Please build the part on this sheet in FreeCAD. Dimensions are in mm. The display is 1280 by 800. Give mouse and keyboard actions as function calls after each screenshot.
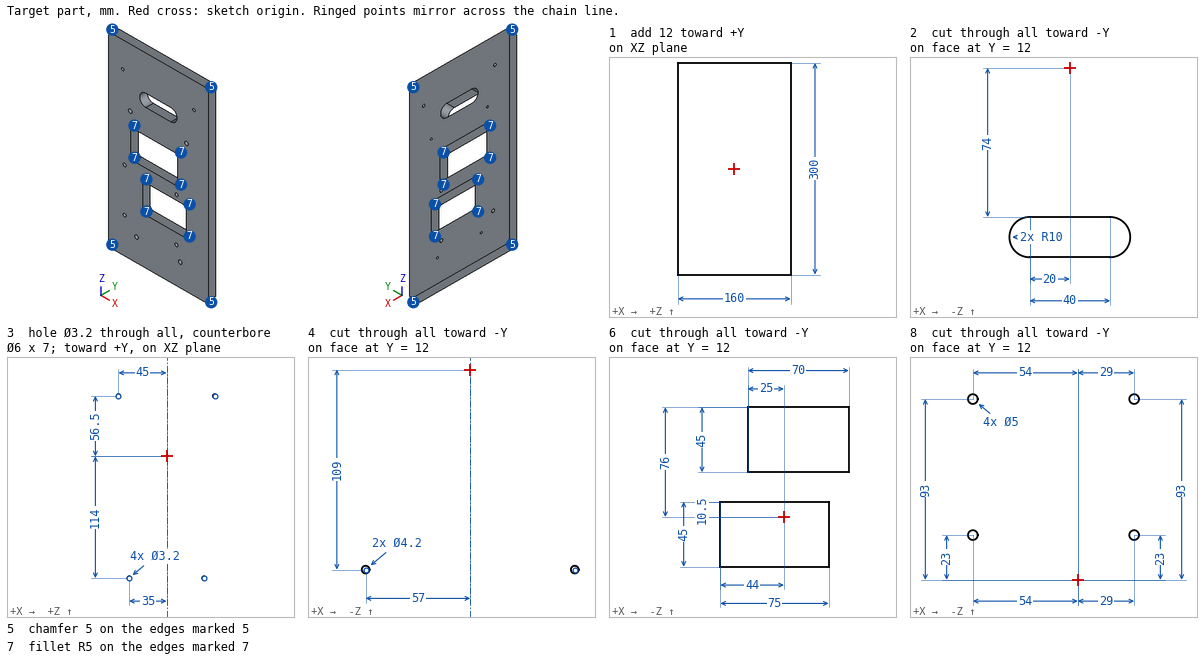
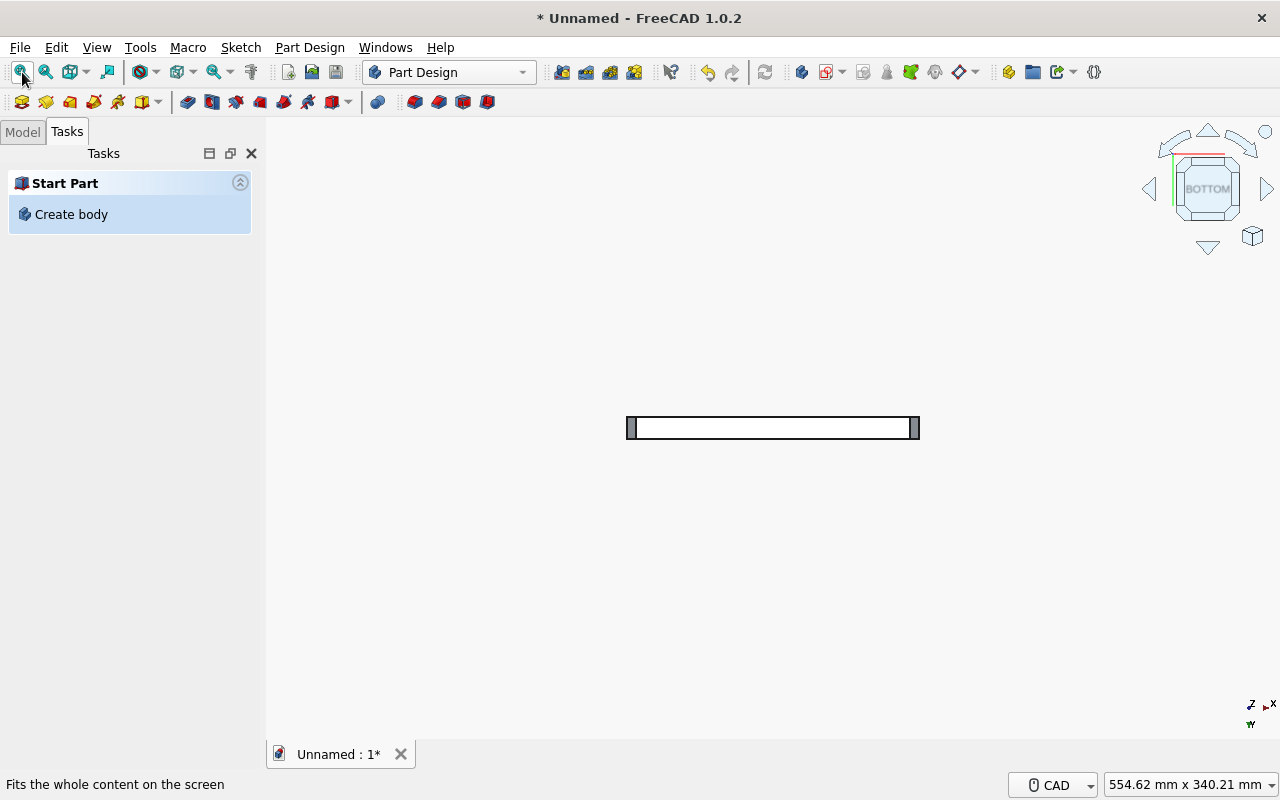
click(22, 72)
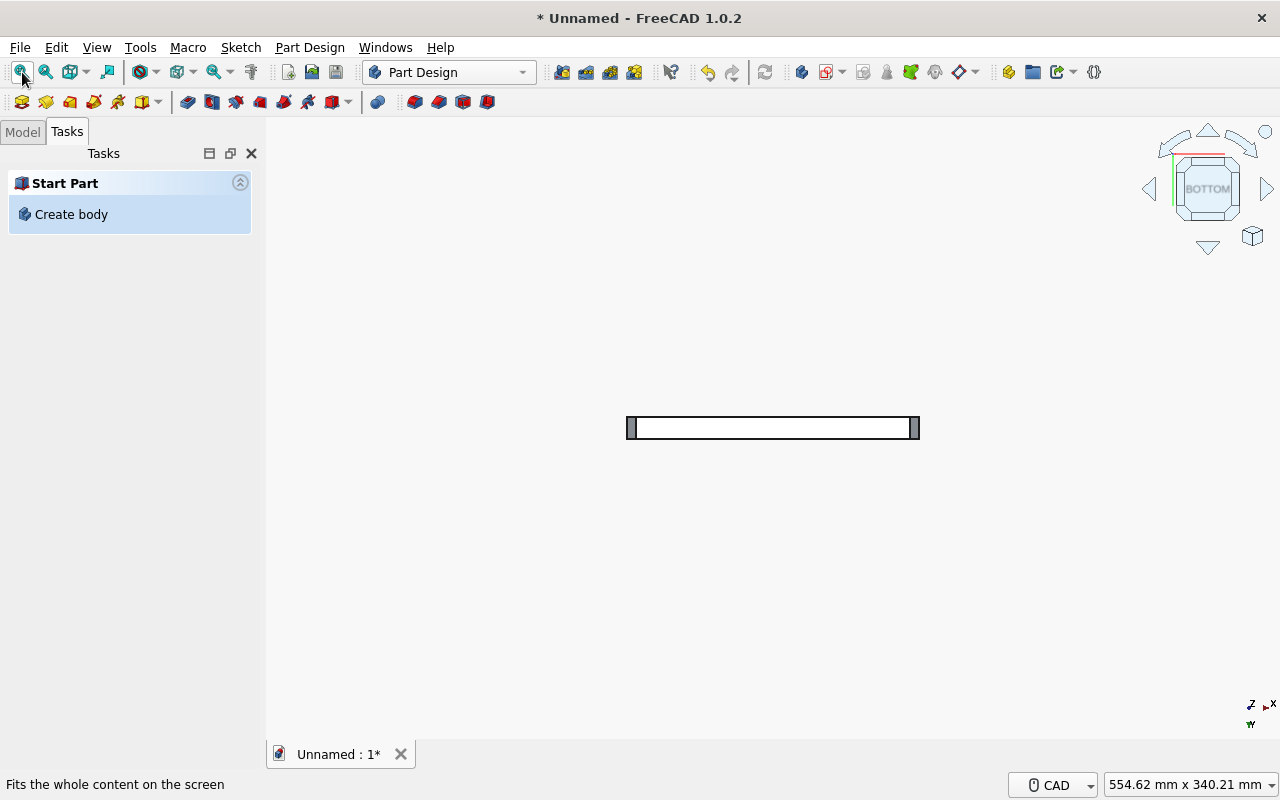
scroll(830, 427, up, 4)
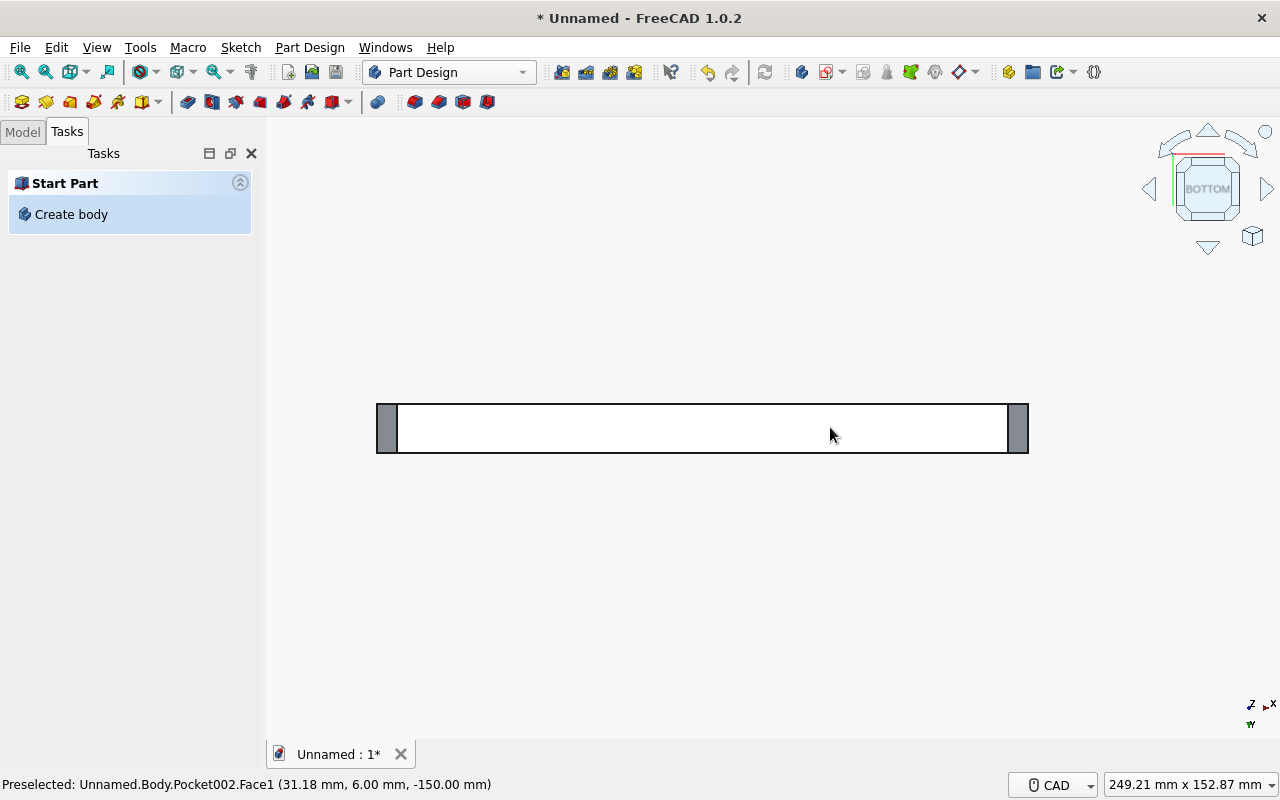
click(22, 72)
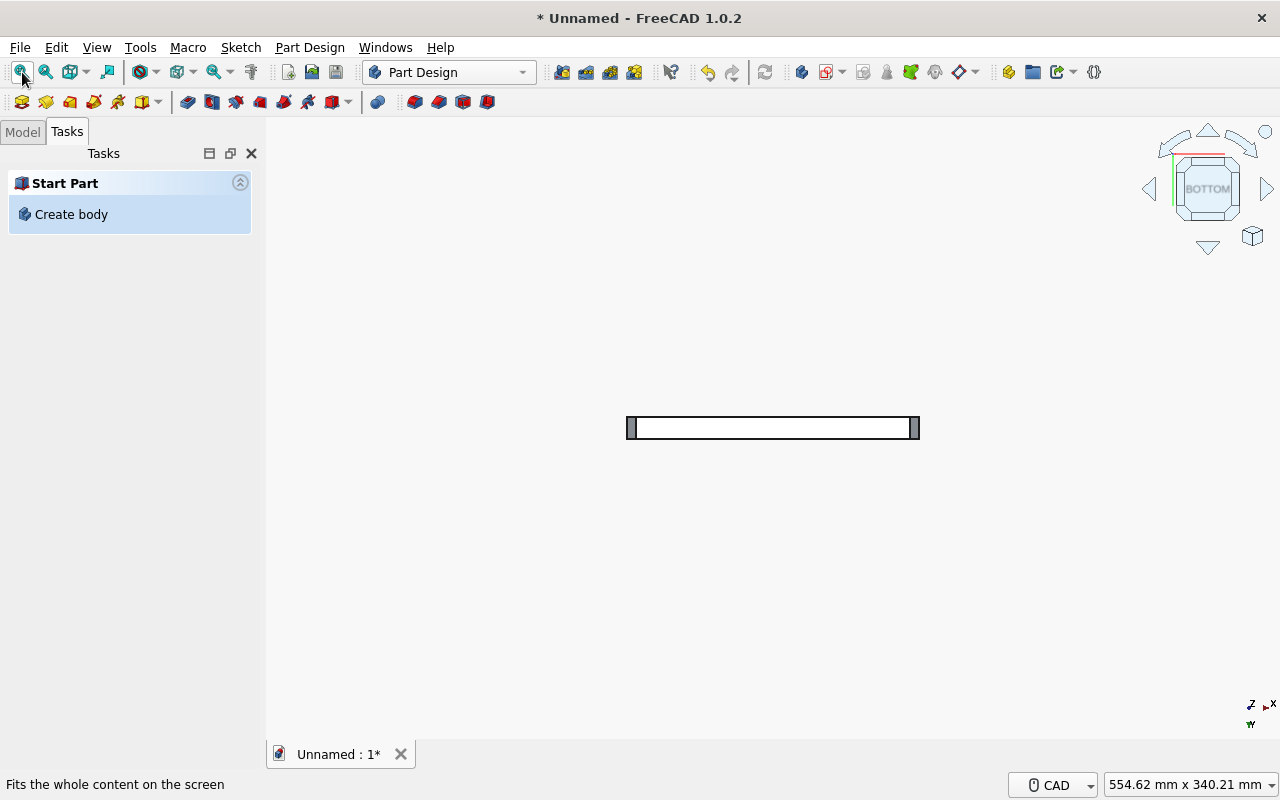
key(4)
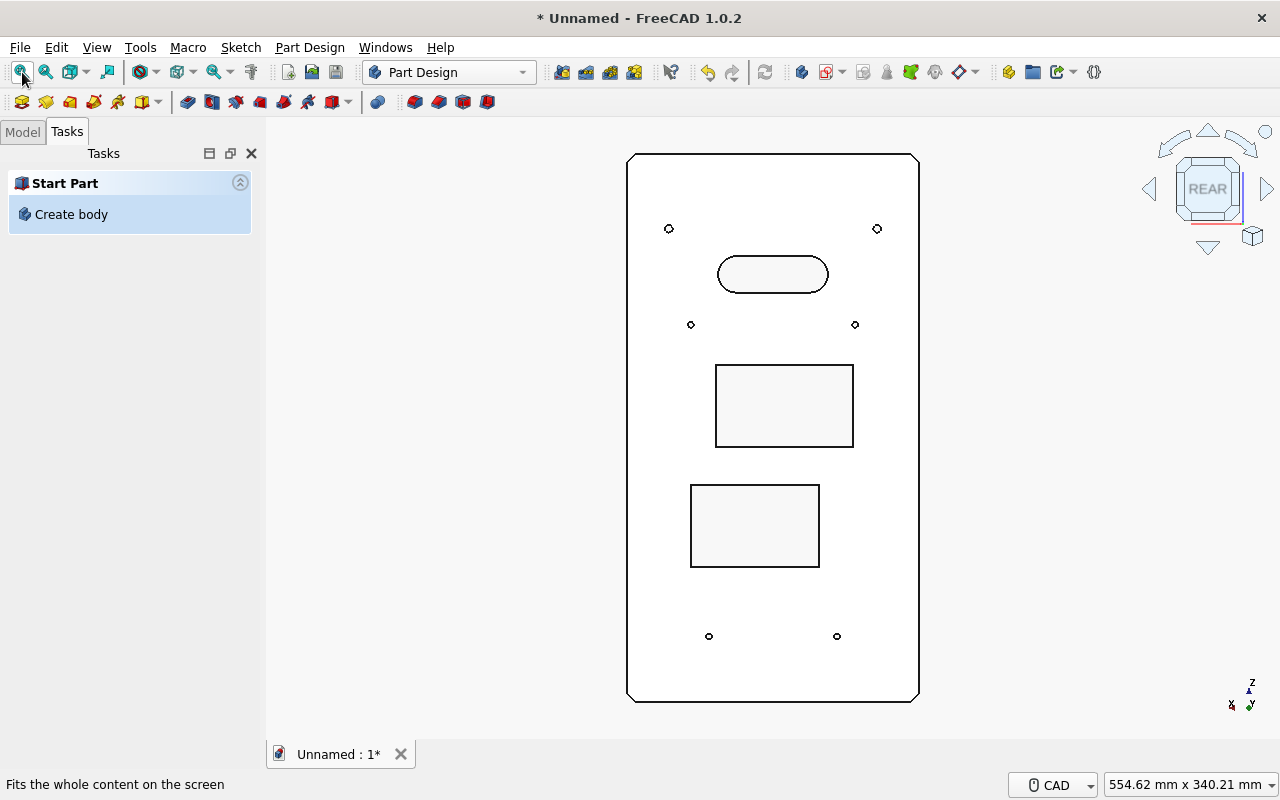
scroll(716, 446, up, 4)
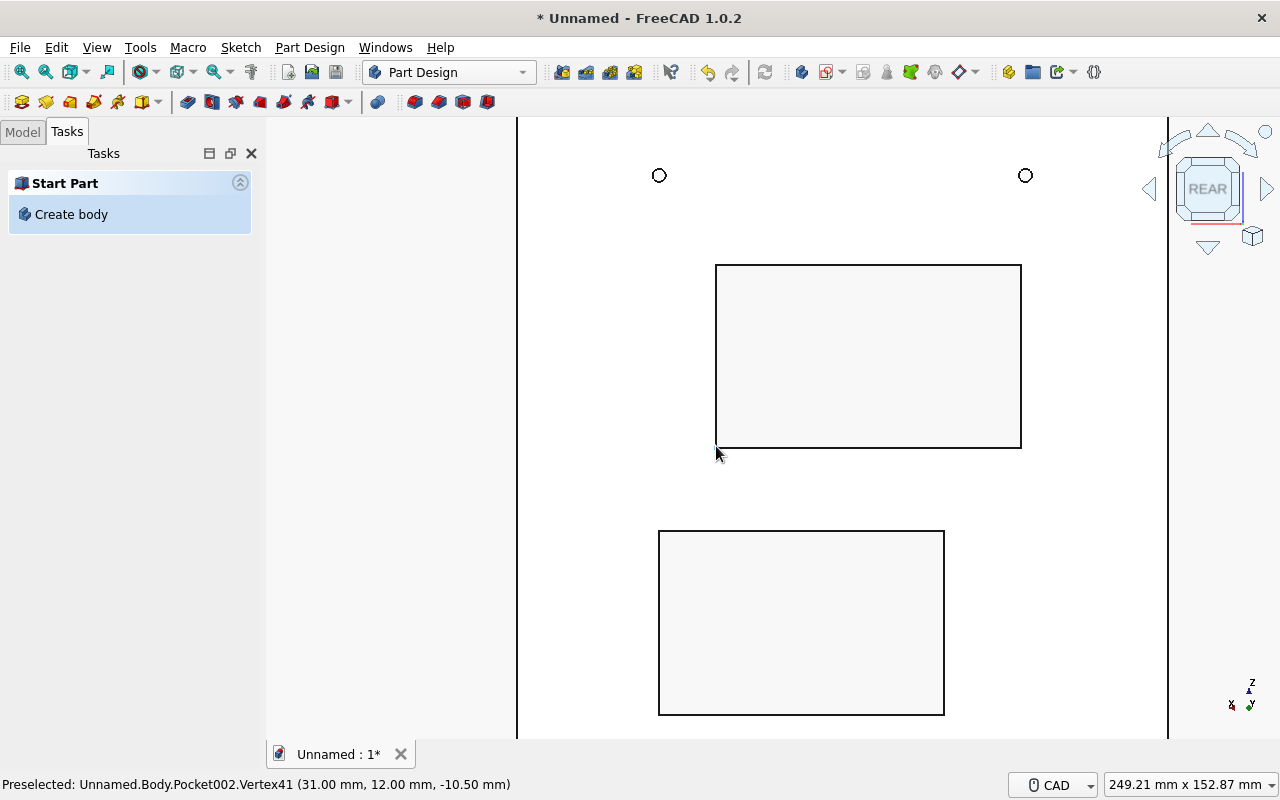
click(22, 72)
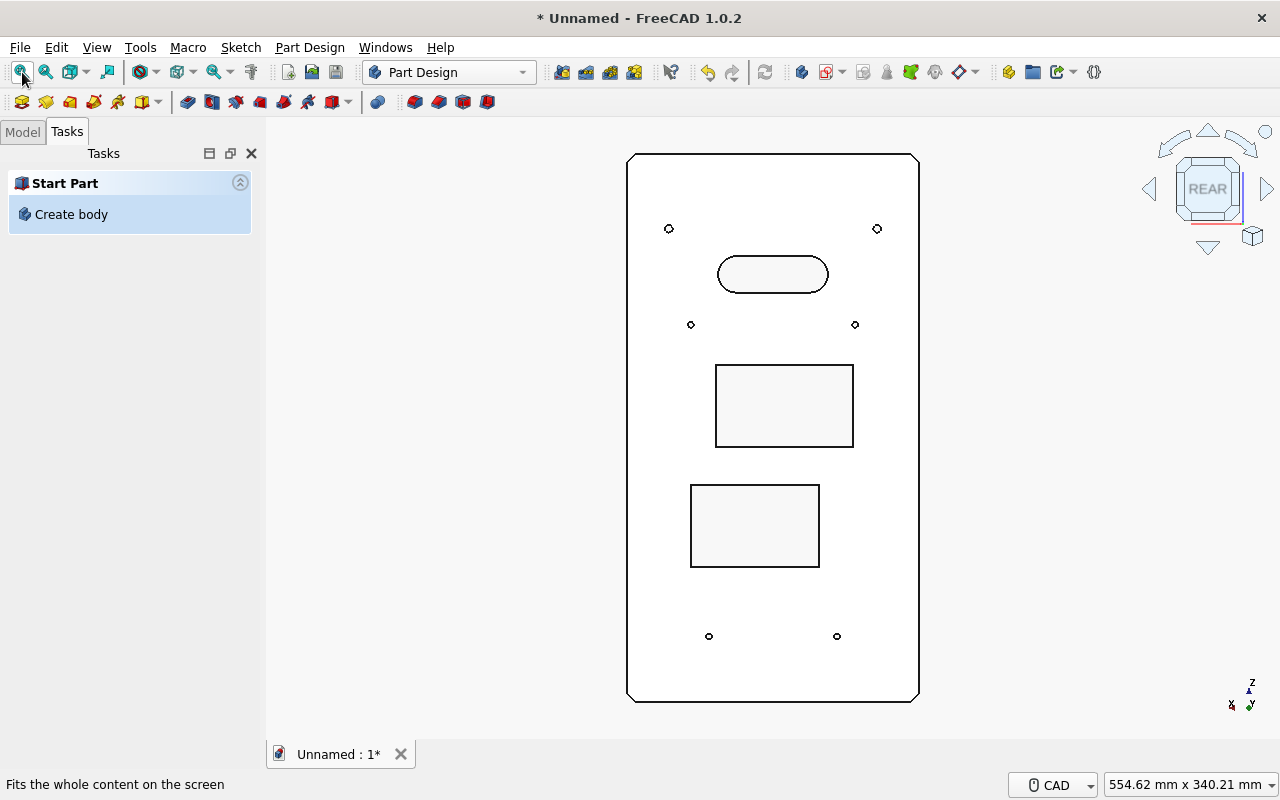
key(6)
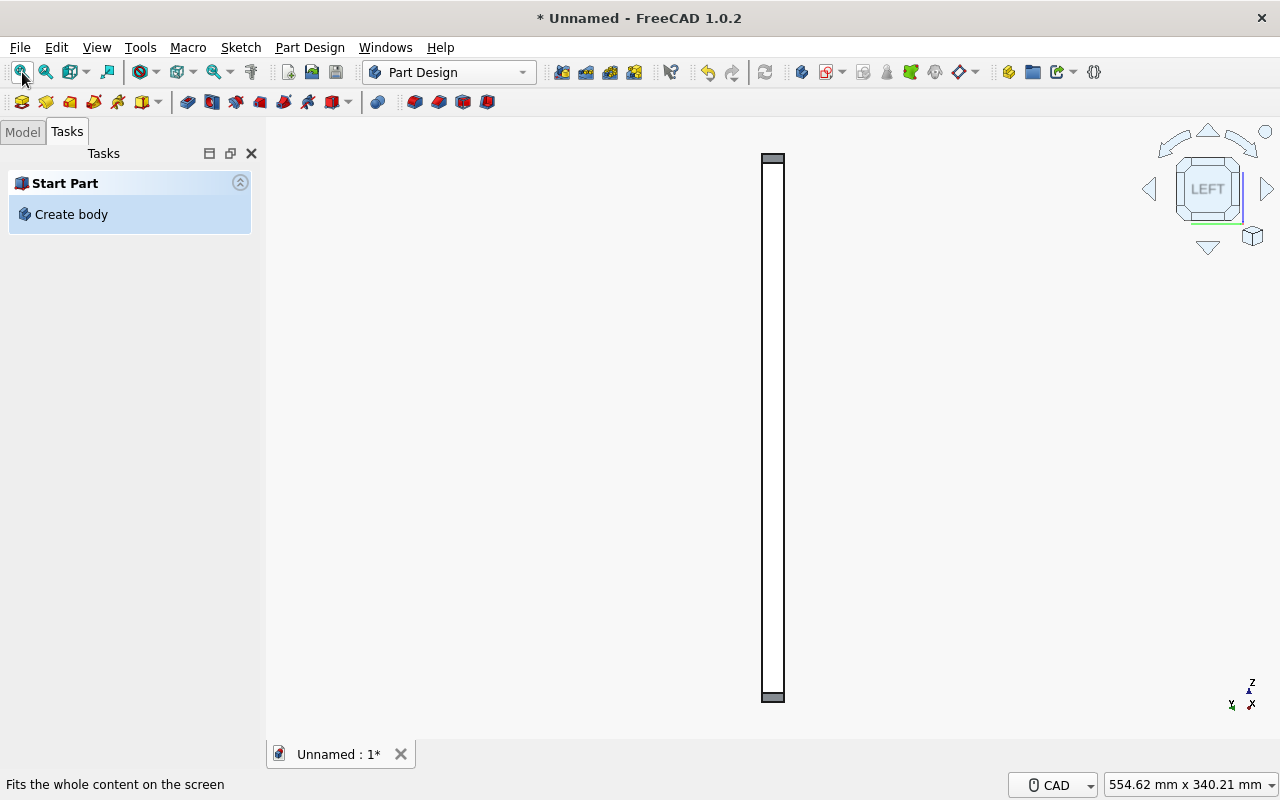
scroll(773, 446, up, 4)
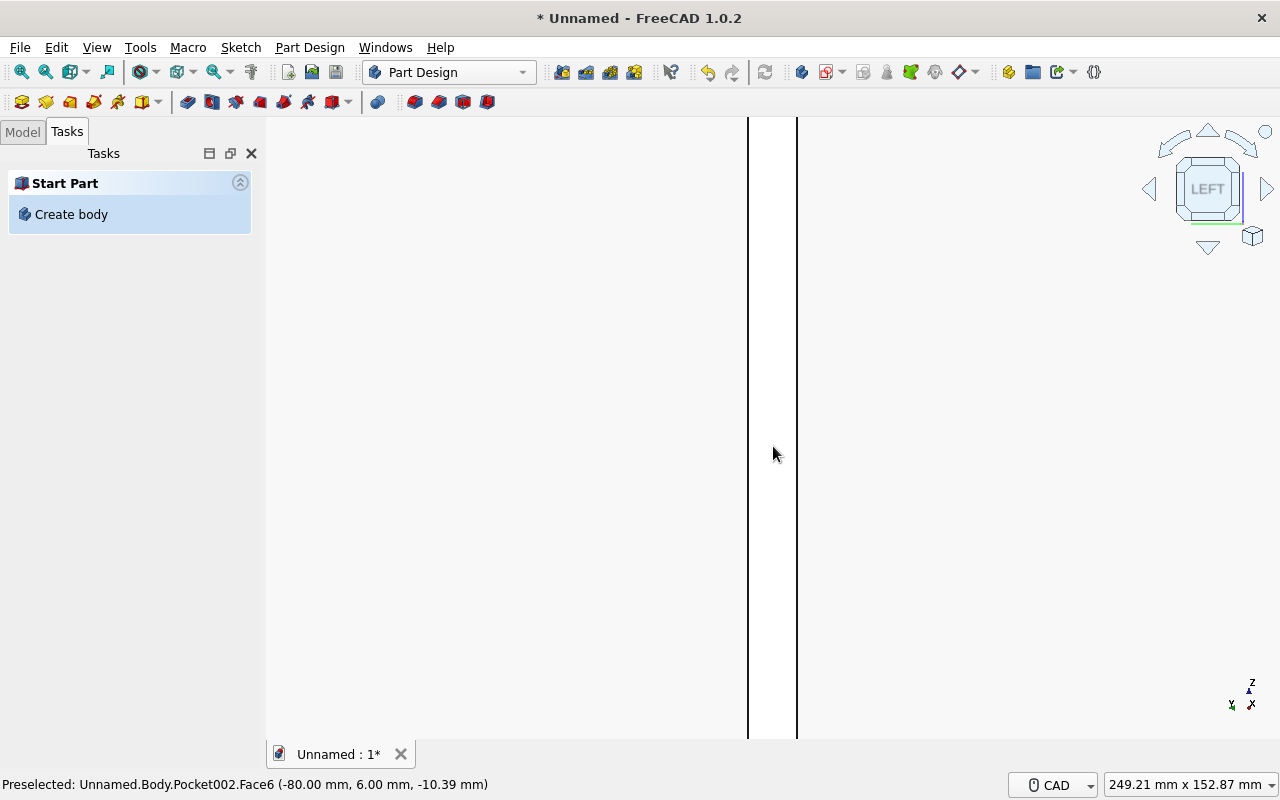
click(22, 72)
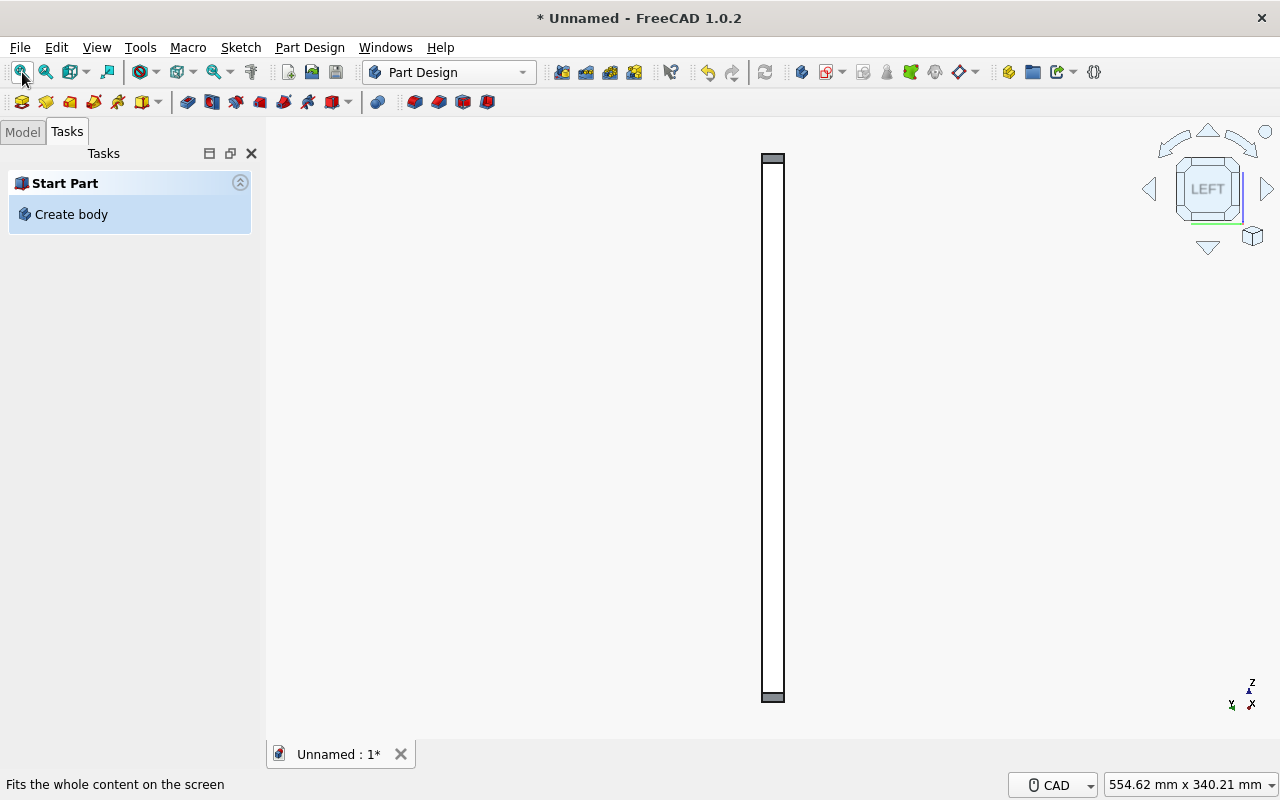
key(v)
key(3)